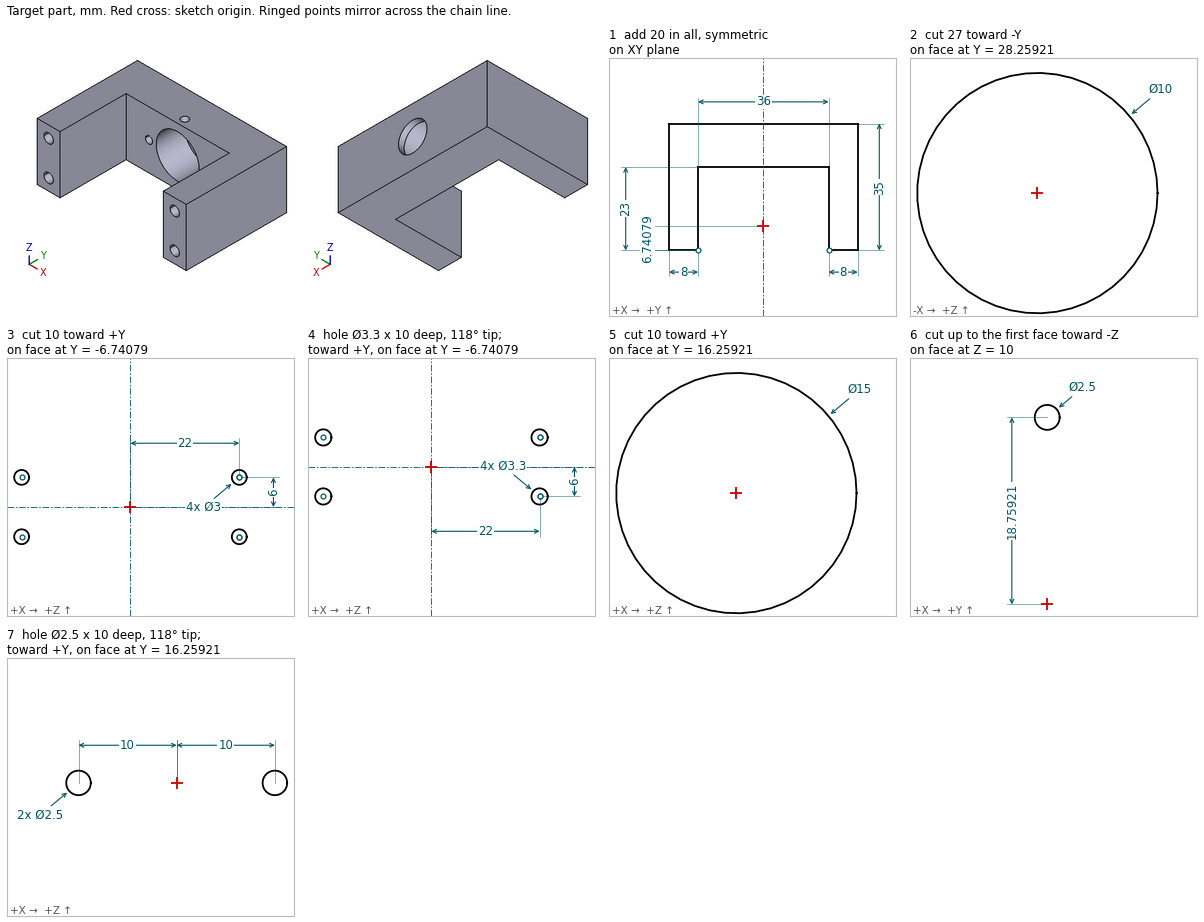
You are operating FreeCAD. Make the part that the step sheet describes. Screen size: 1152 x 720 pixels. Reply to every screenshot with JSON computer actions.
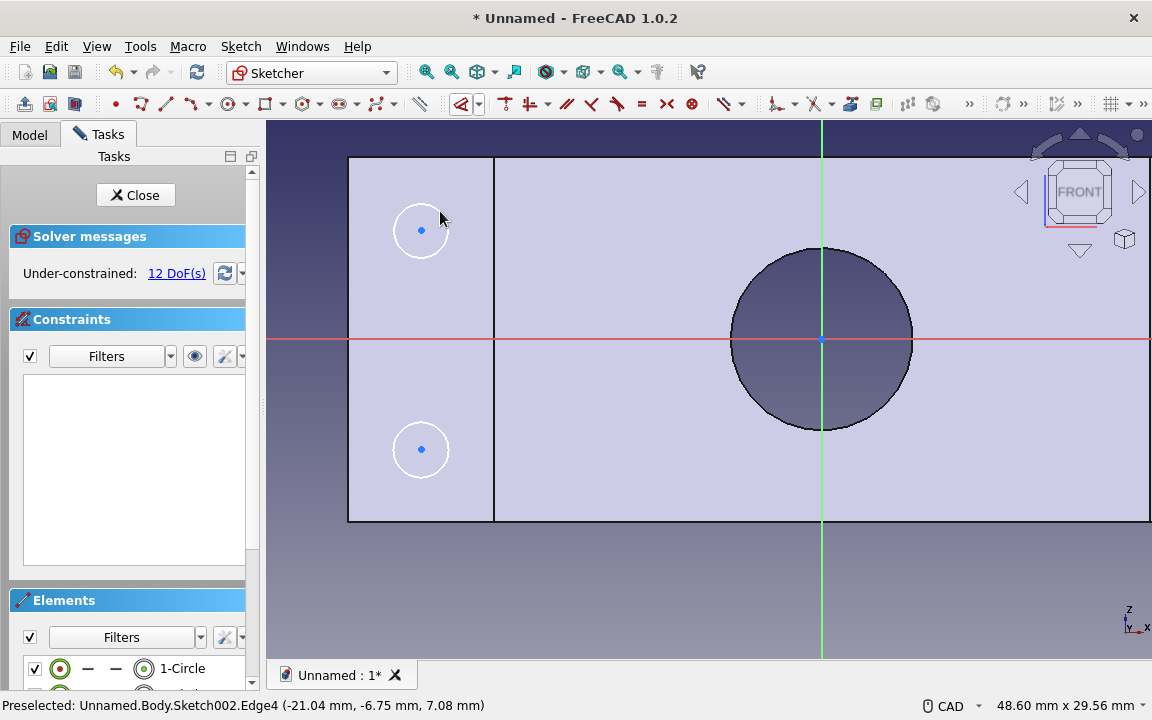
{"action": "scroll", "coordinate": [420, 451], "scroll_direction": "down", "scroll_amount": 3}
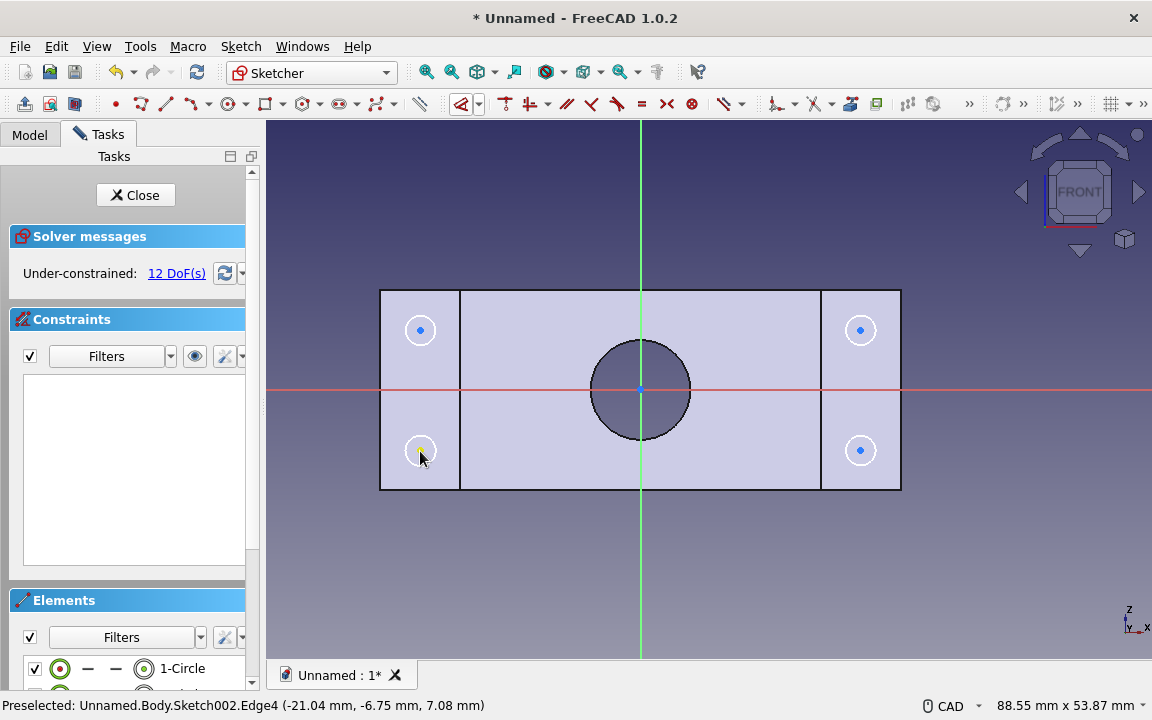
{"action": "left_click", "coordinate": [871, 320]}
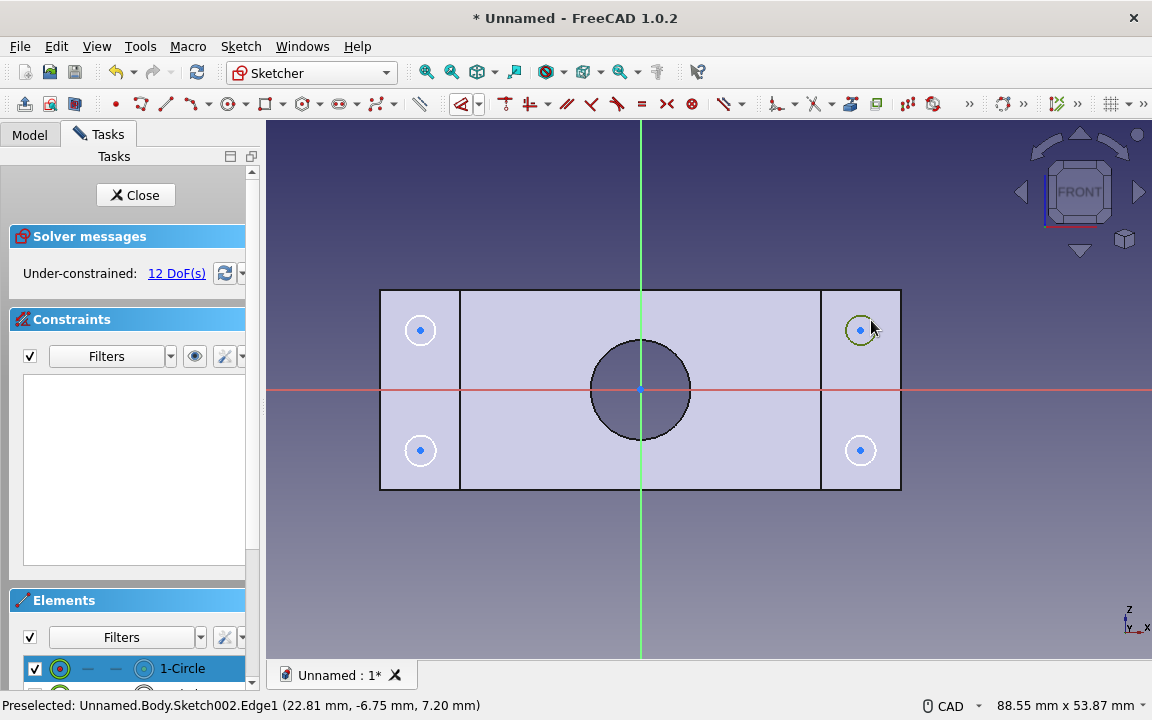
{"action": "left_click", "coordinate": [871, 440]}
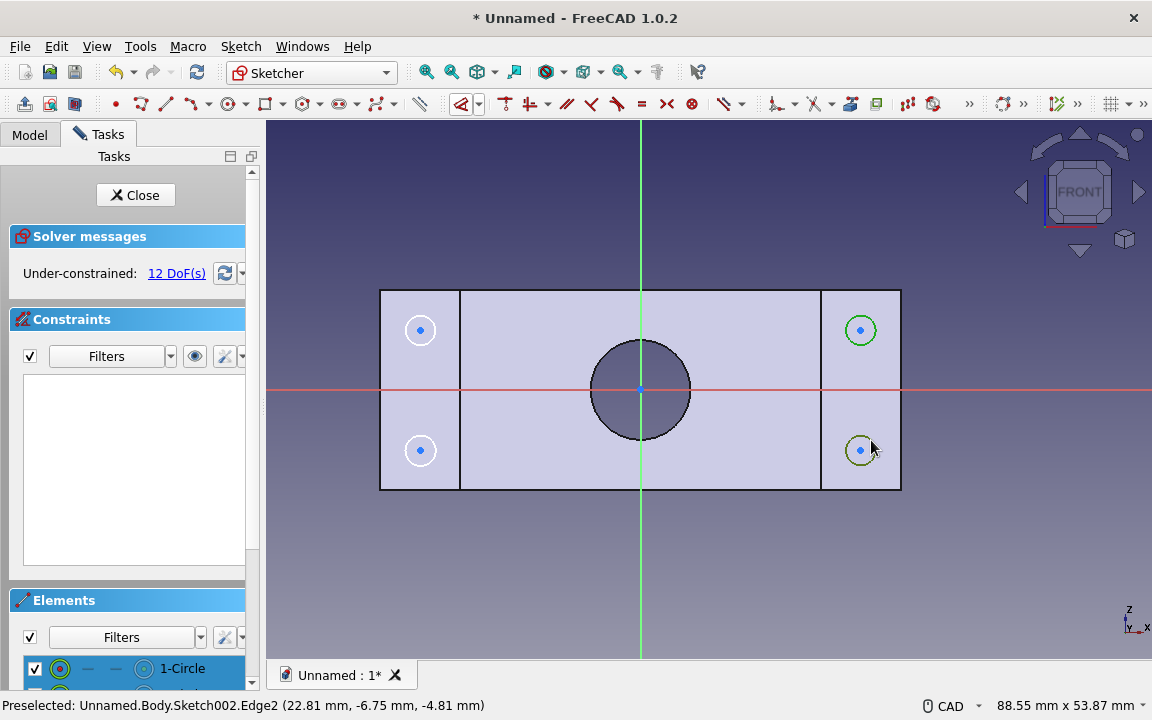
{"action": "left_click", "coordinate": [431, 440]}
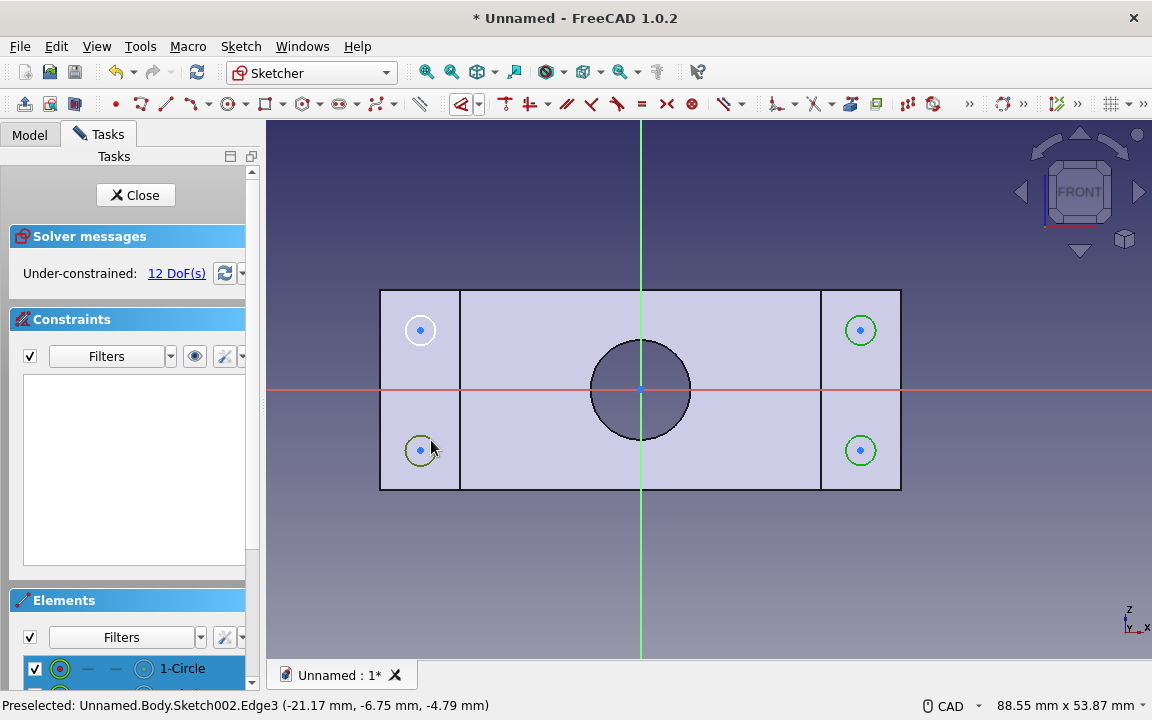
{"action": "left_click", "coordinate": [431, 320]}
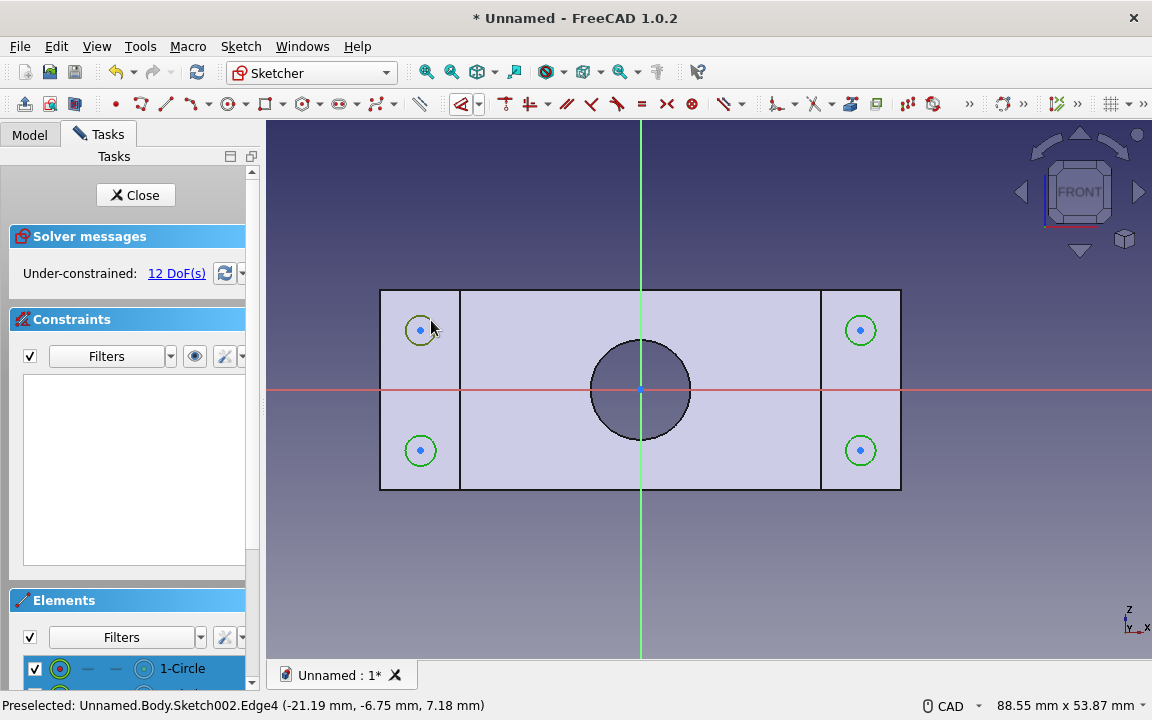
{"action": "left_click", "coordinate": [642, 104]}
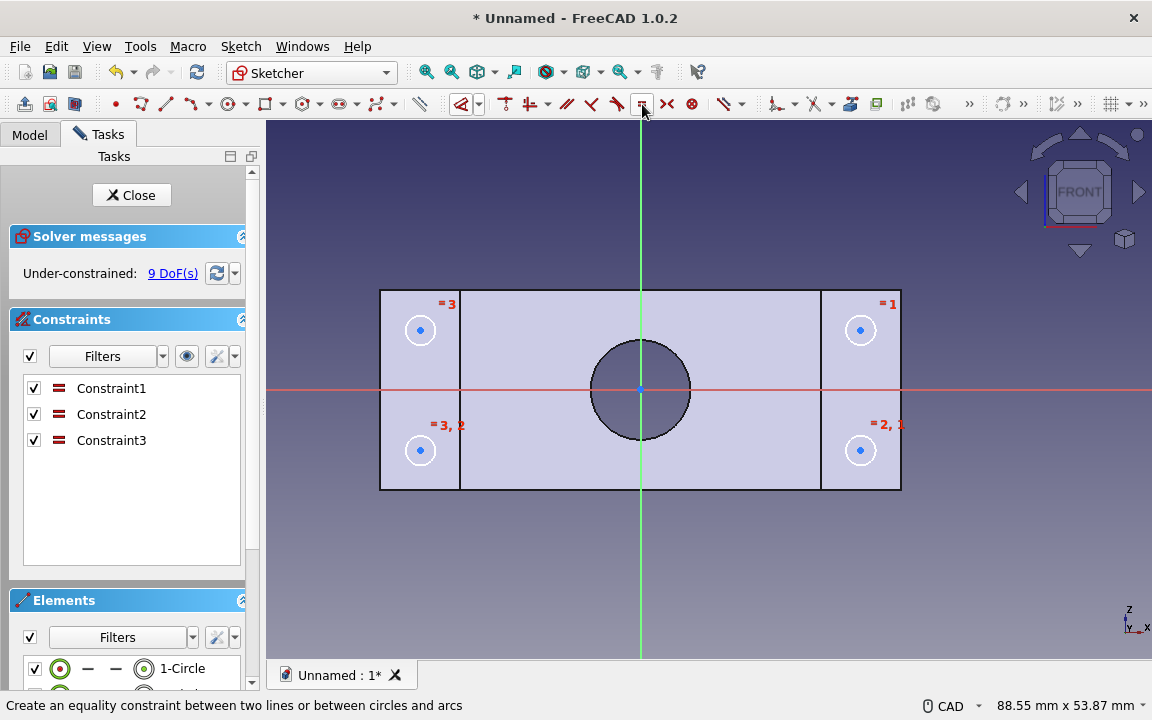
{"action": "left_click", "coordinate": [861, 330]}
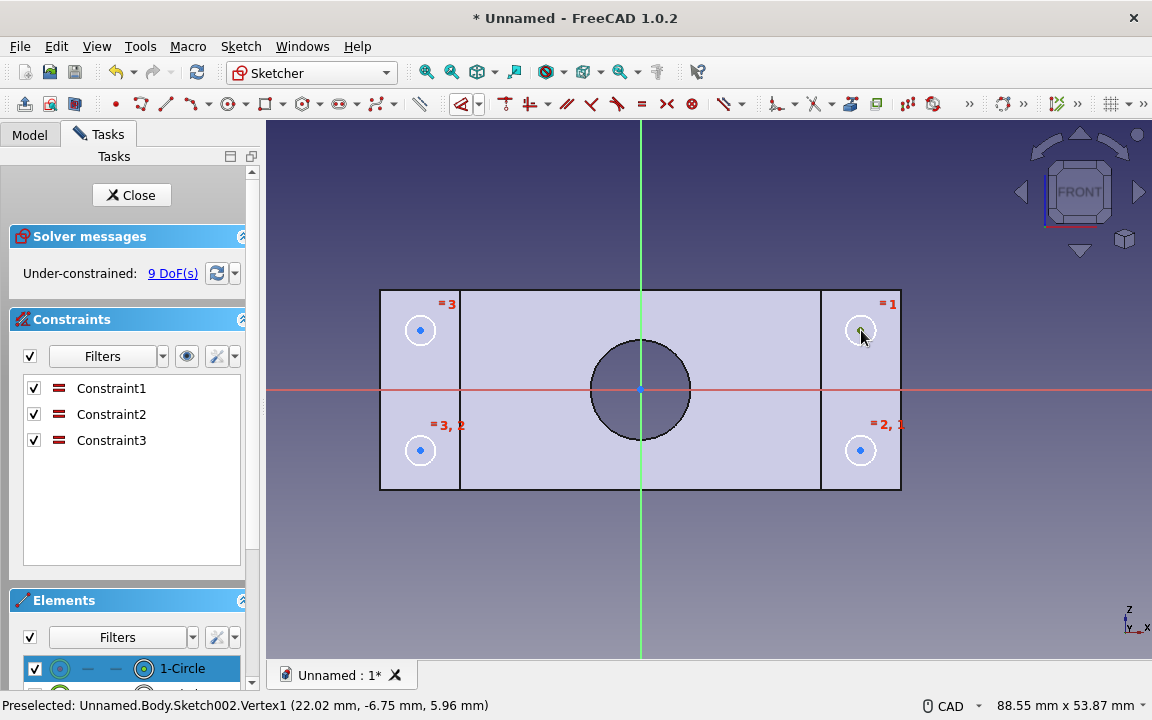
{"action": "left_click", "coordinate": [861, 451]}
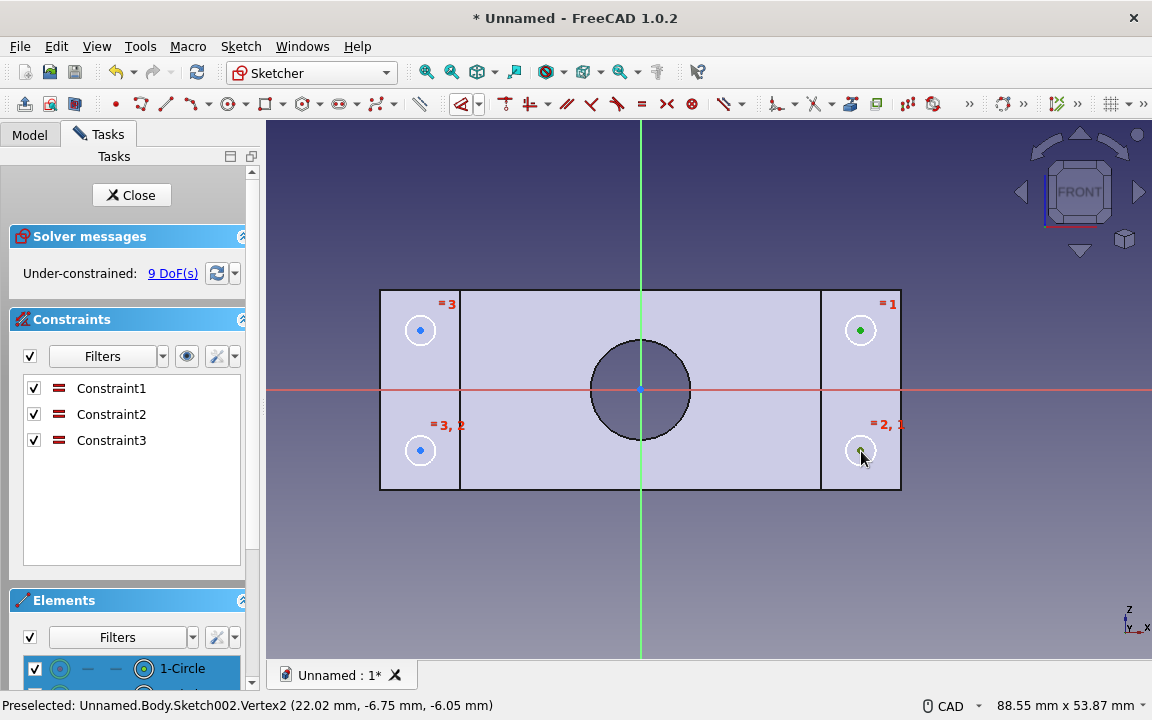
{"action": "left_click", "coordinate": [344, 390]}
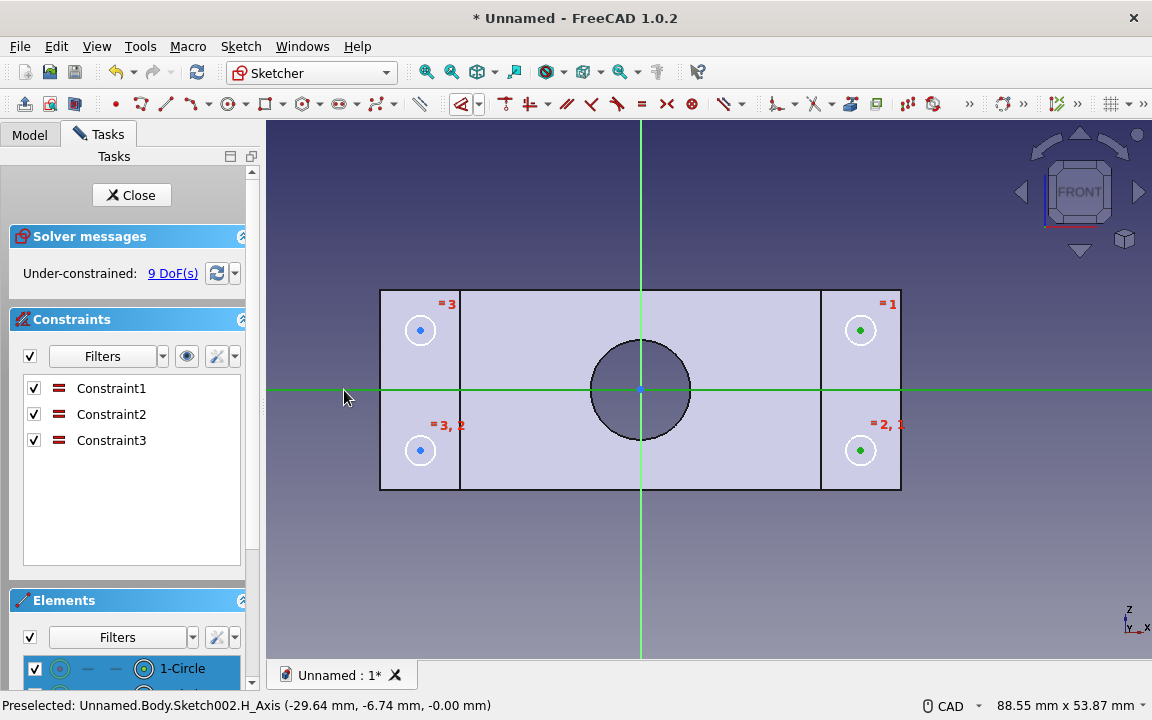
{"action": "key", "text": "s"}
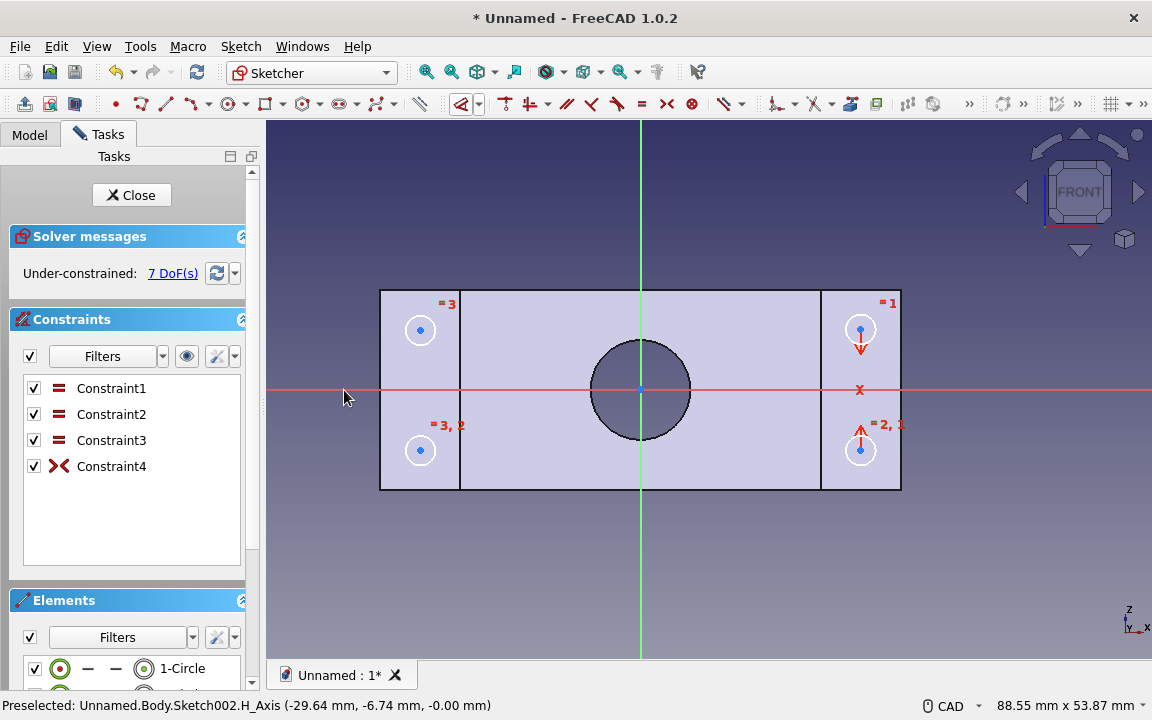
{"action": "left_click", "coordinate": [861, 451]}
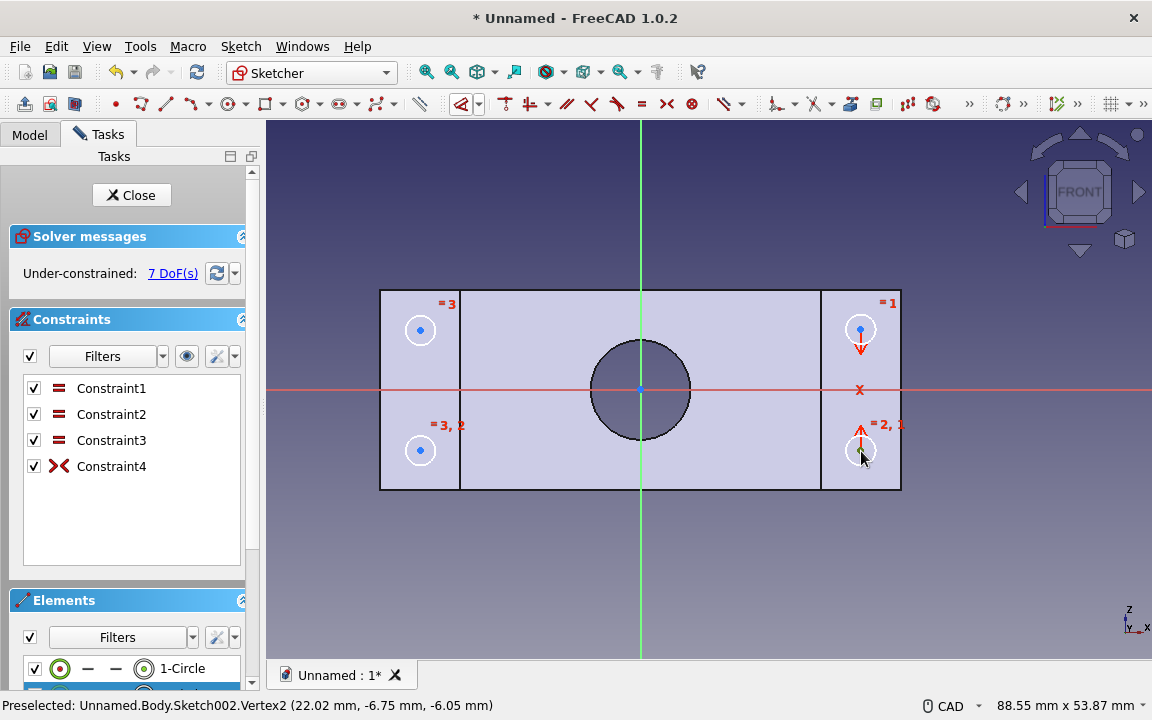
{"action": "left_click", "coordinate": [421, 451]}